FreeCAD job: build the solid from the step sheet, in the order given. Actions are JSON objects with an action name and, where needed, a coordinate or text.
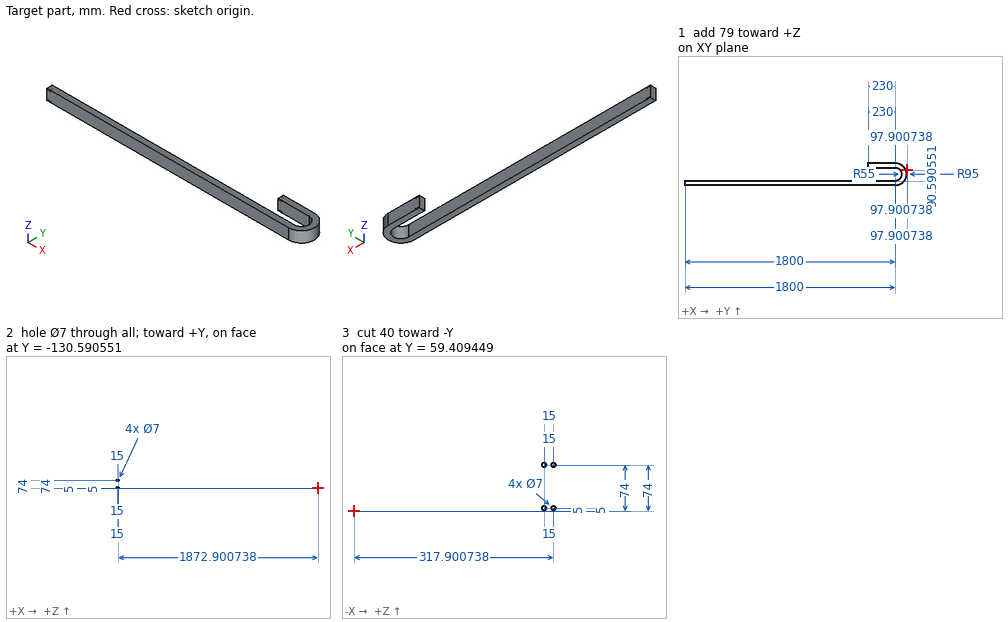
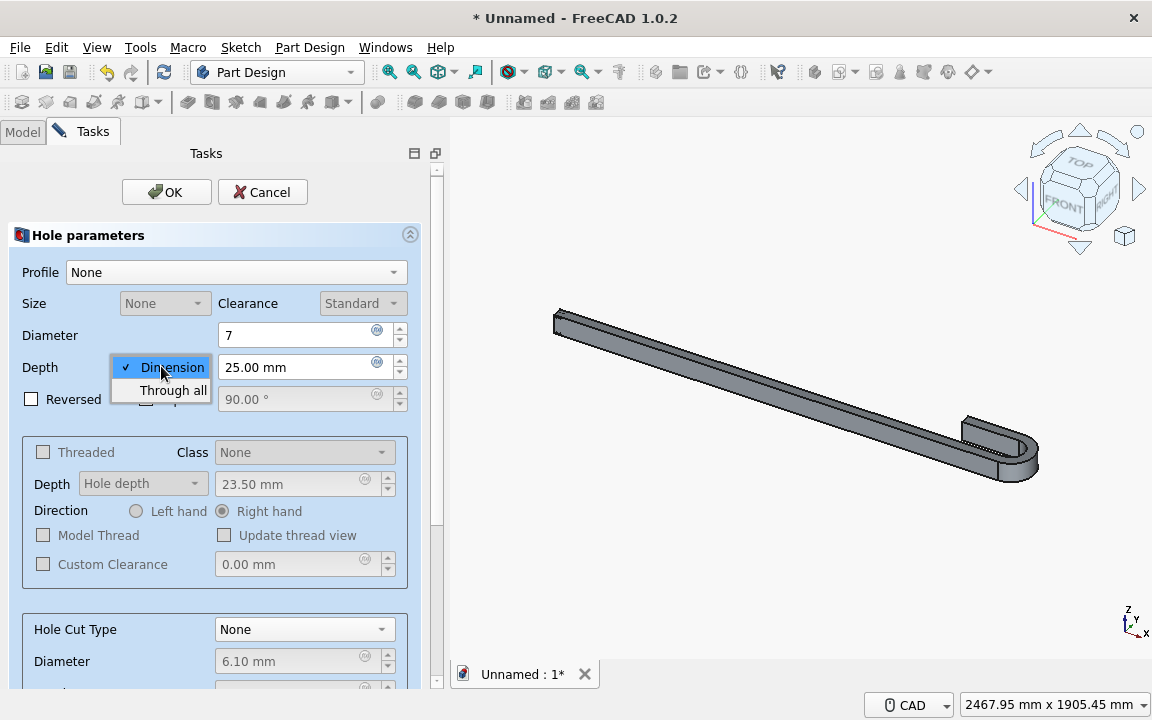
{"action": "left_click", "coordinate": [160, 390]}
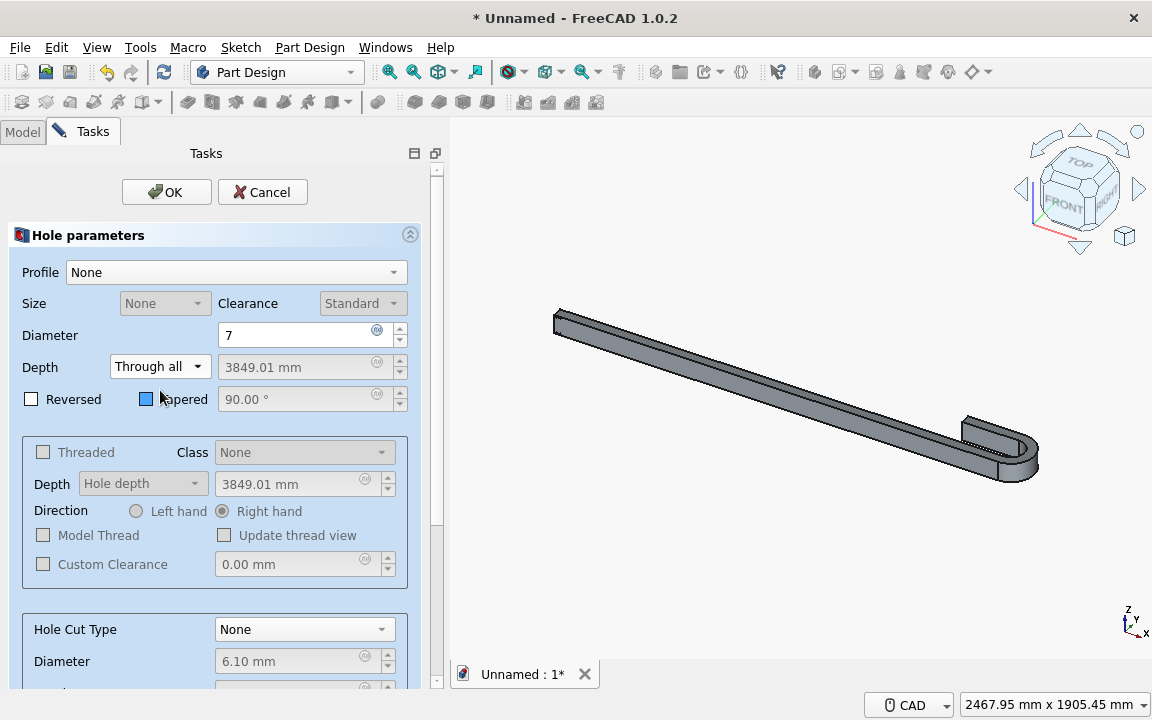
{"action": "left_click", "coordinate": [167, 192]}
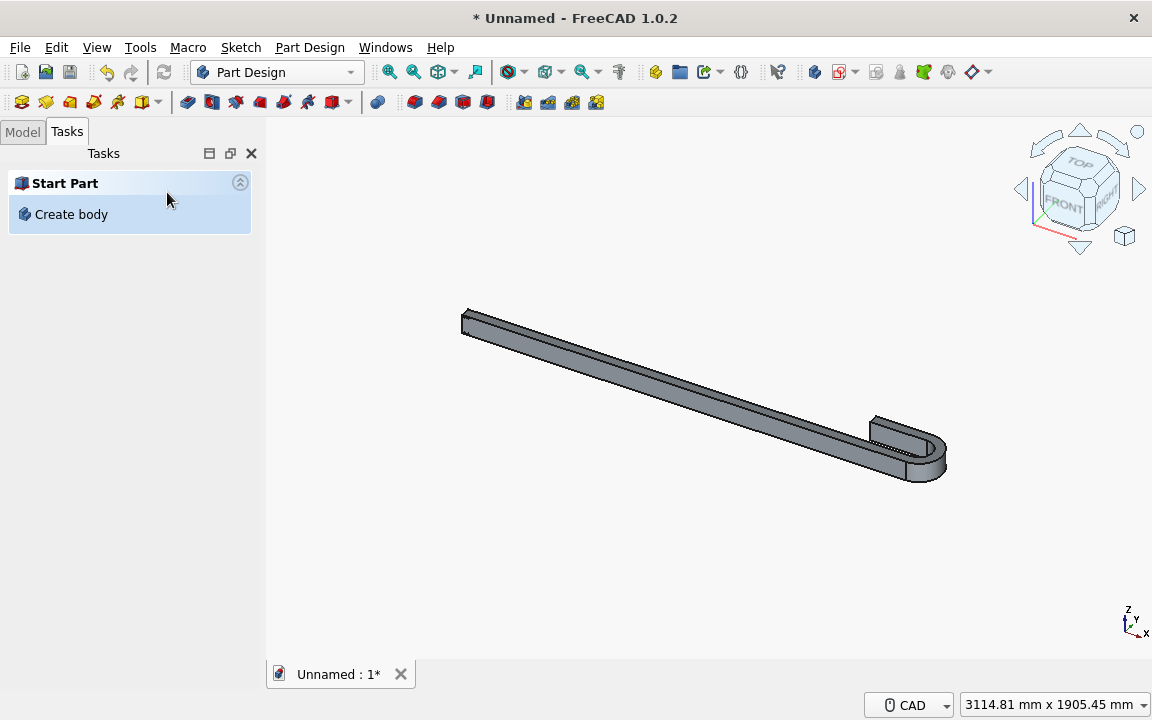
{"action": "key", "text": "4"}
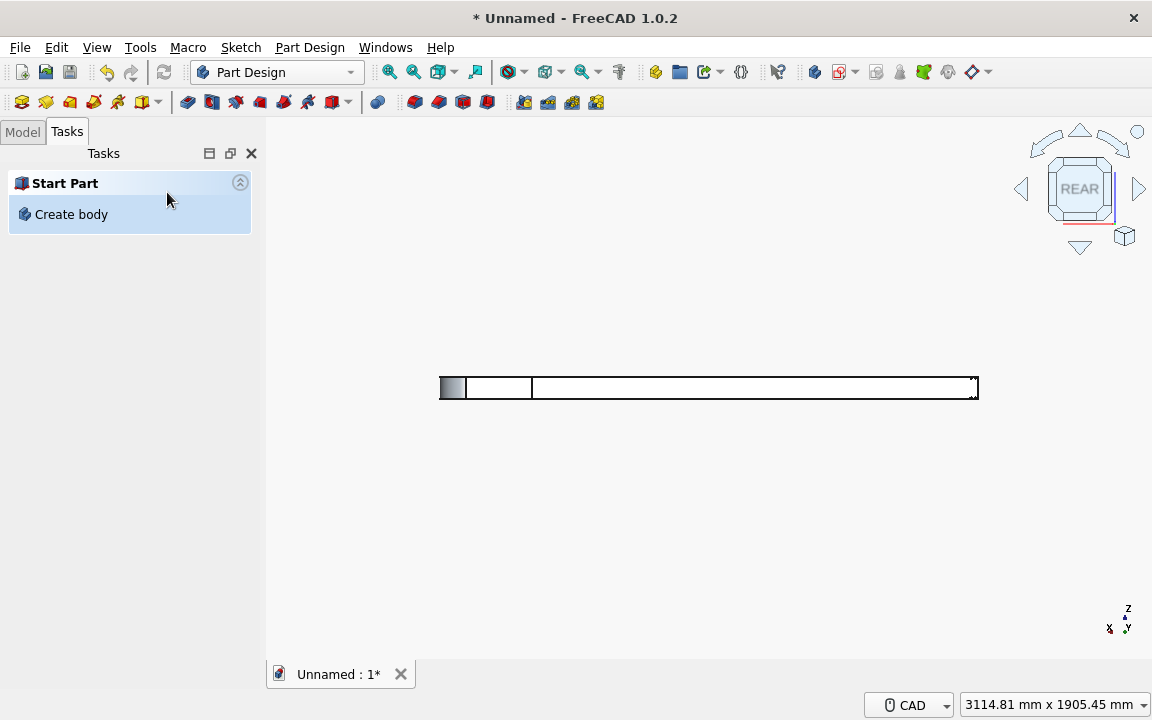
{"action": "left_click", "coordinate": [480, 387]}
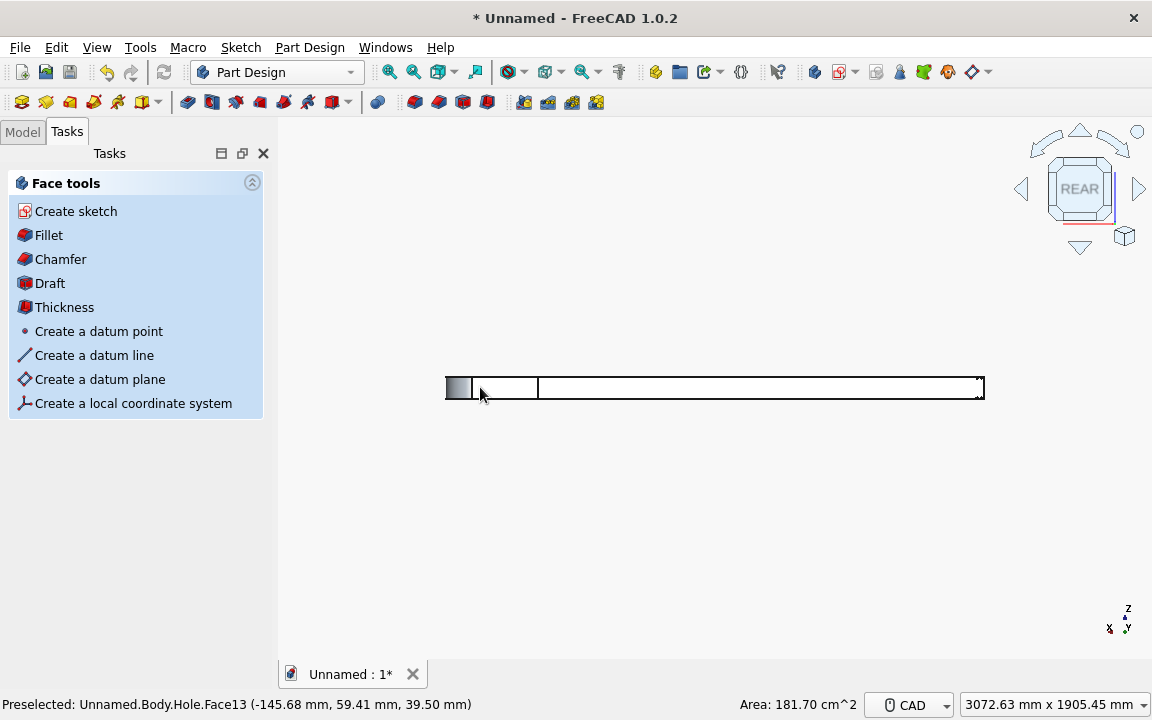
{"action": "left_click", "coordinate": [840, 72]}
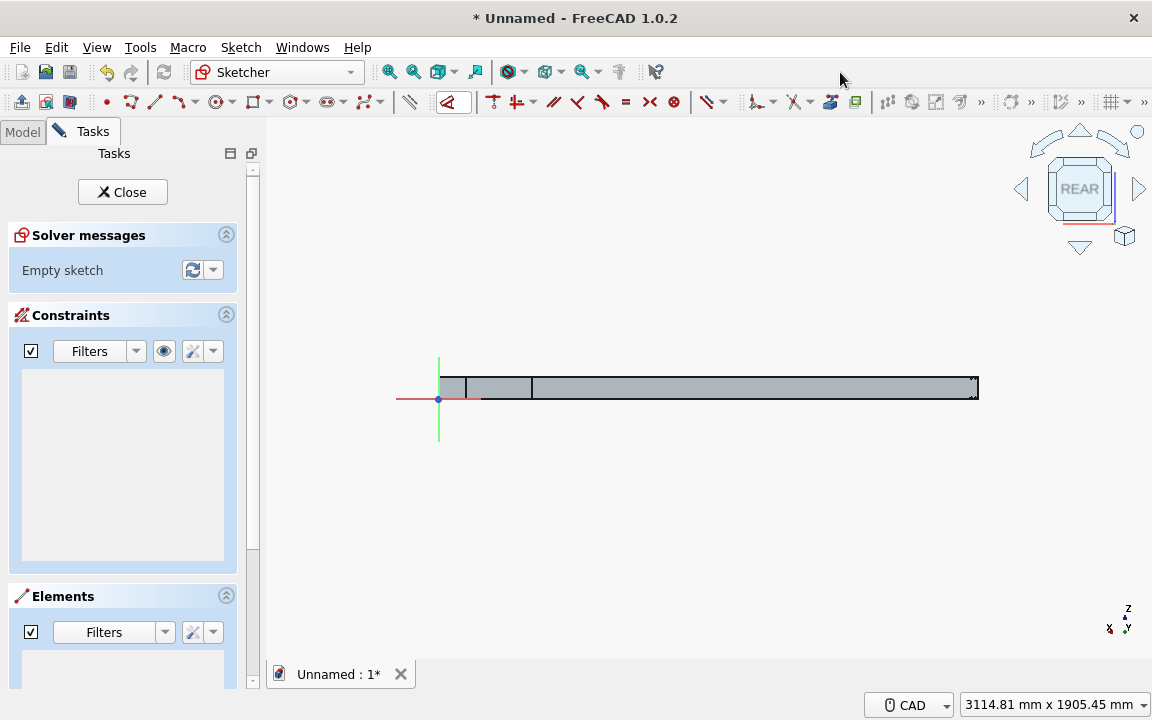
{"action": "scroll", "coordinate": [519, 388], "scroll_direction": "up", "scroll_amount": 14}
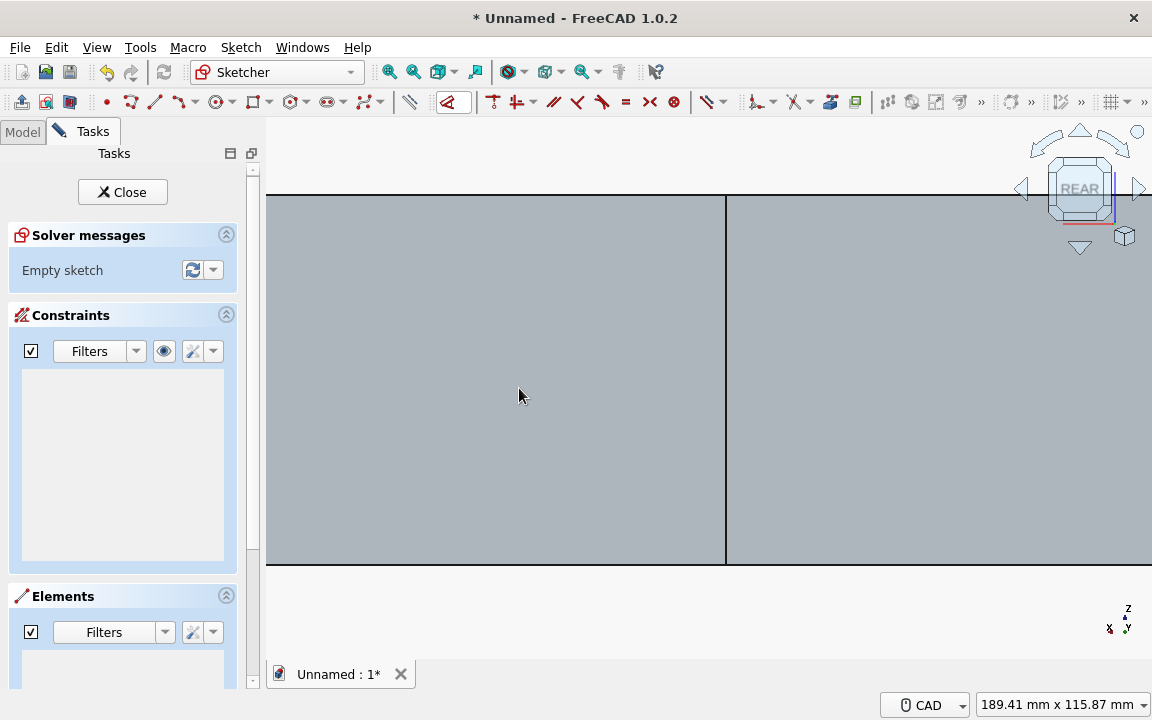
{"action": "key", "text": "g c"}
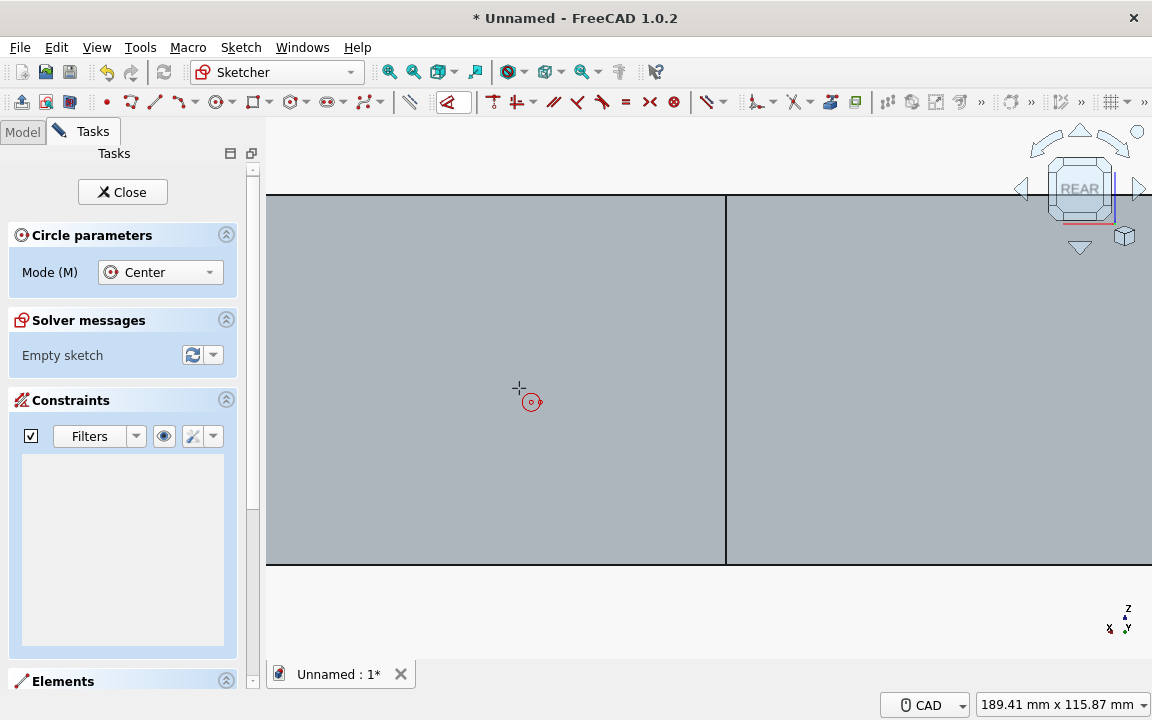
{"action": "scroll", "coordinate": [679, 542], "scroll_direction": "up", "scroll_amount": 2}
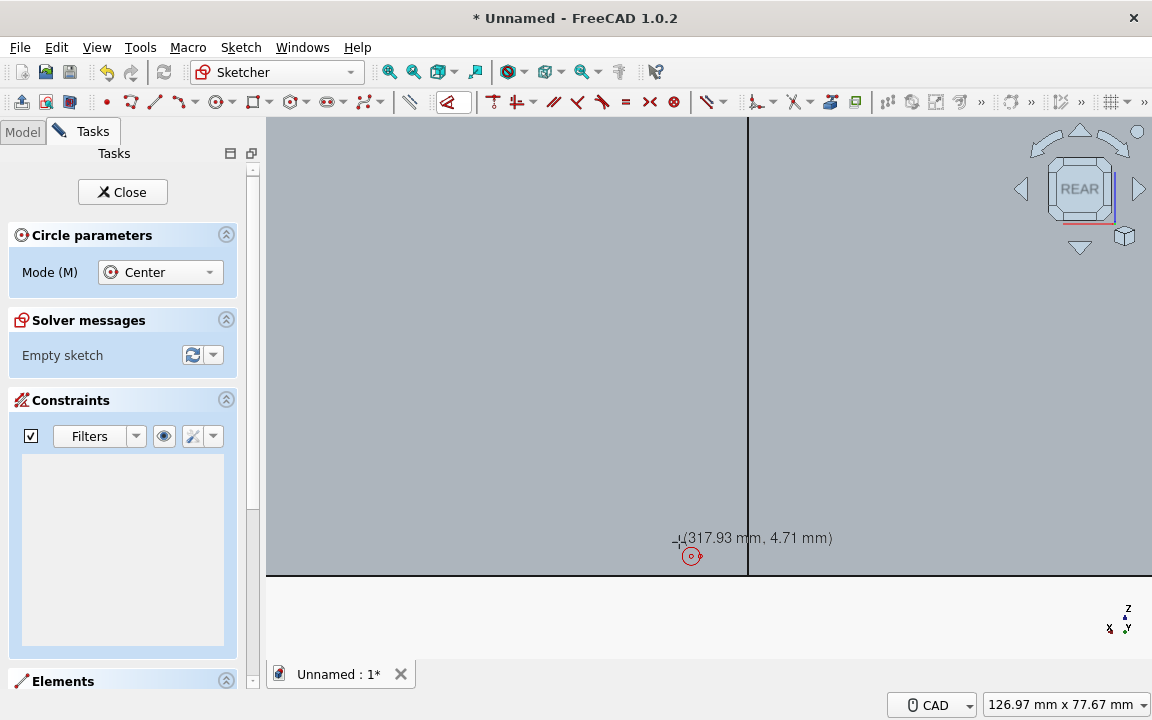
{"action": "left_click", "coordinate": [679, 541]}
{"action": "left_click", "coordinate": [696, 524]}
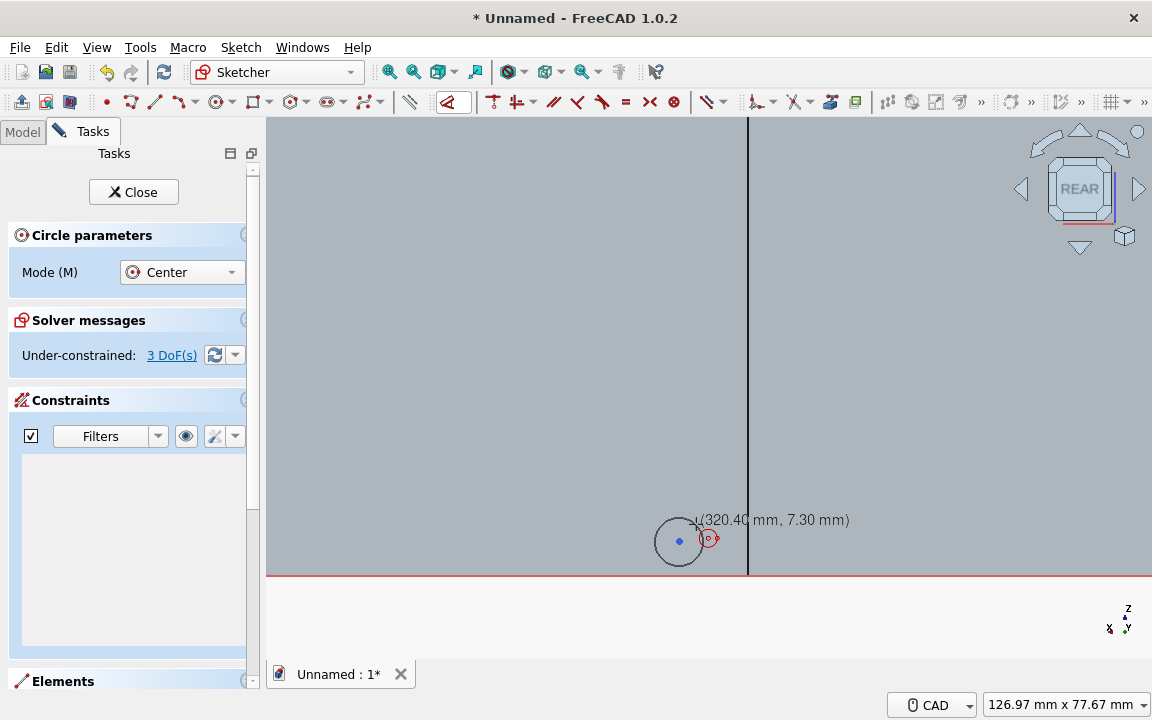
{"action": "left_click", "coordinate": [574, 541]}
{"action": "left_click", "coordinate": [591, 524]}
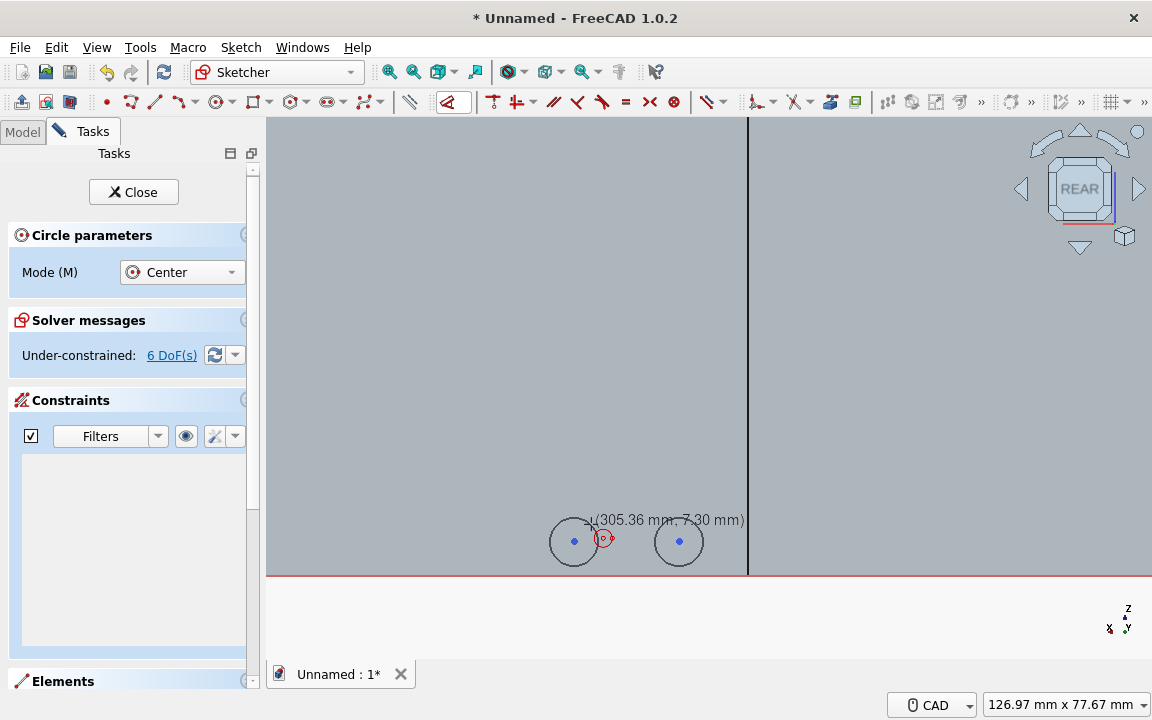
{"action": "scroll", "coordinate": [670, 566], "scroll_direction": "down", "scroll_amount": 2}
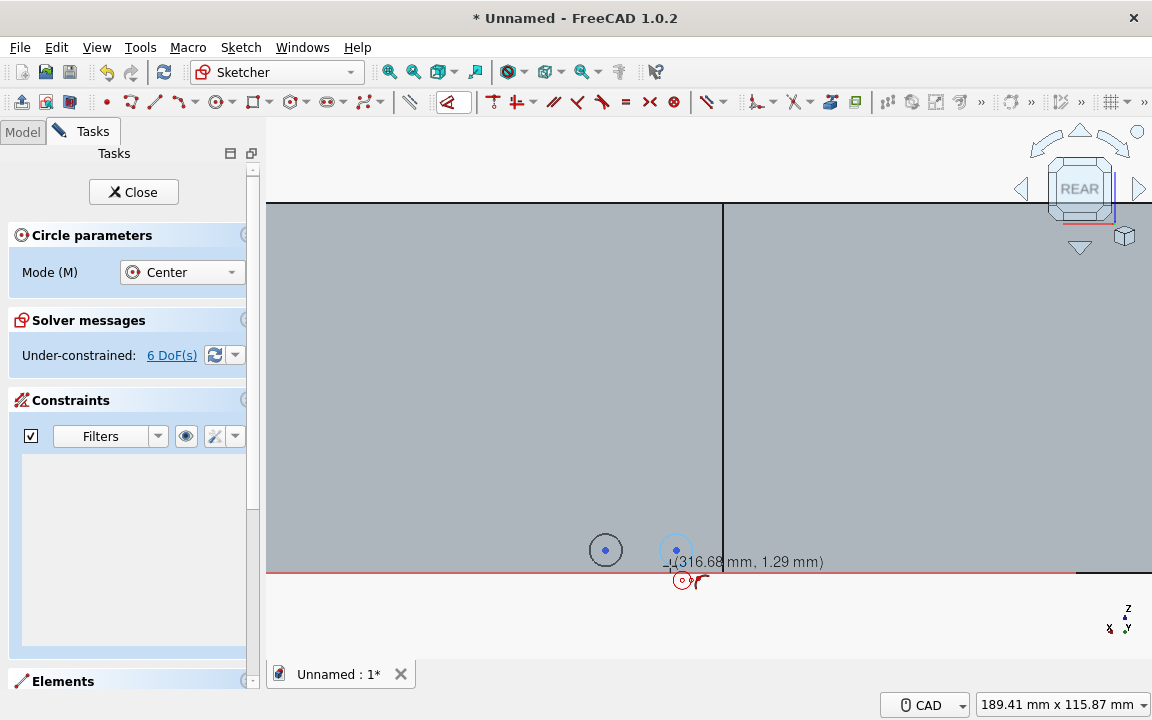
{"action": "scroll", "coordinate": [676, 227], "scroll_direction": "up", "scroll_amount": 2}